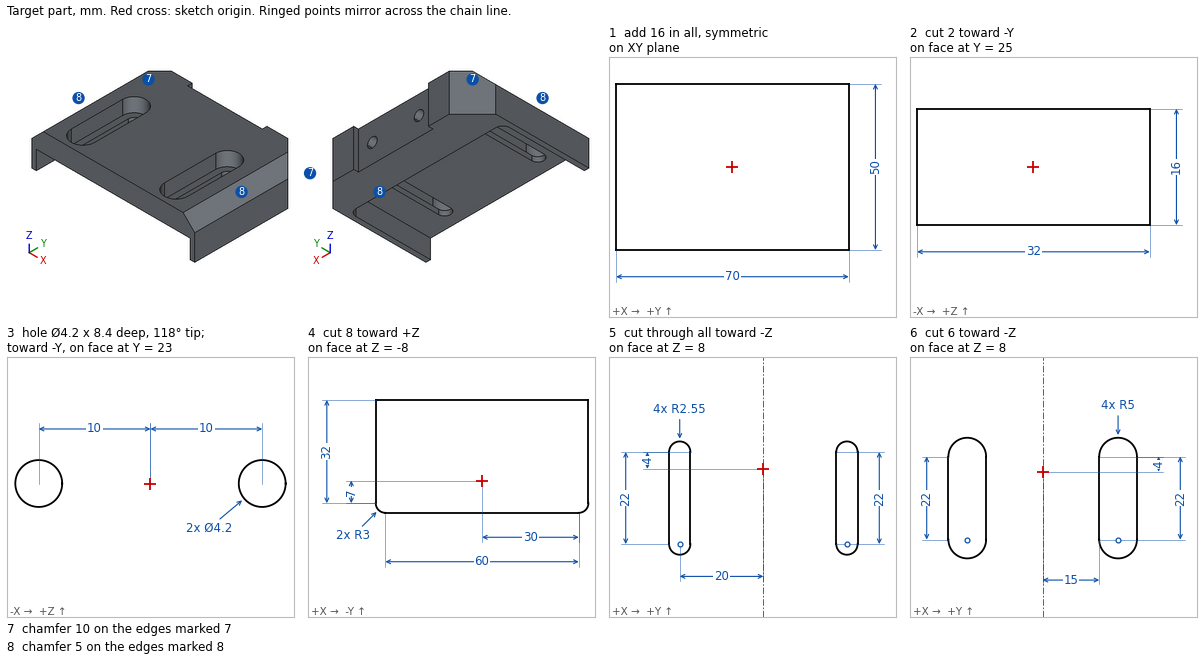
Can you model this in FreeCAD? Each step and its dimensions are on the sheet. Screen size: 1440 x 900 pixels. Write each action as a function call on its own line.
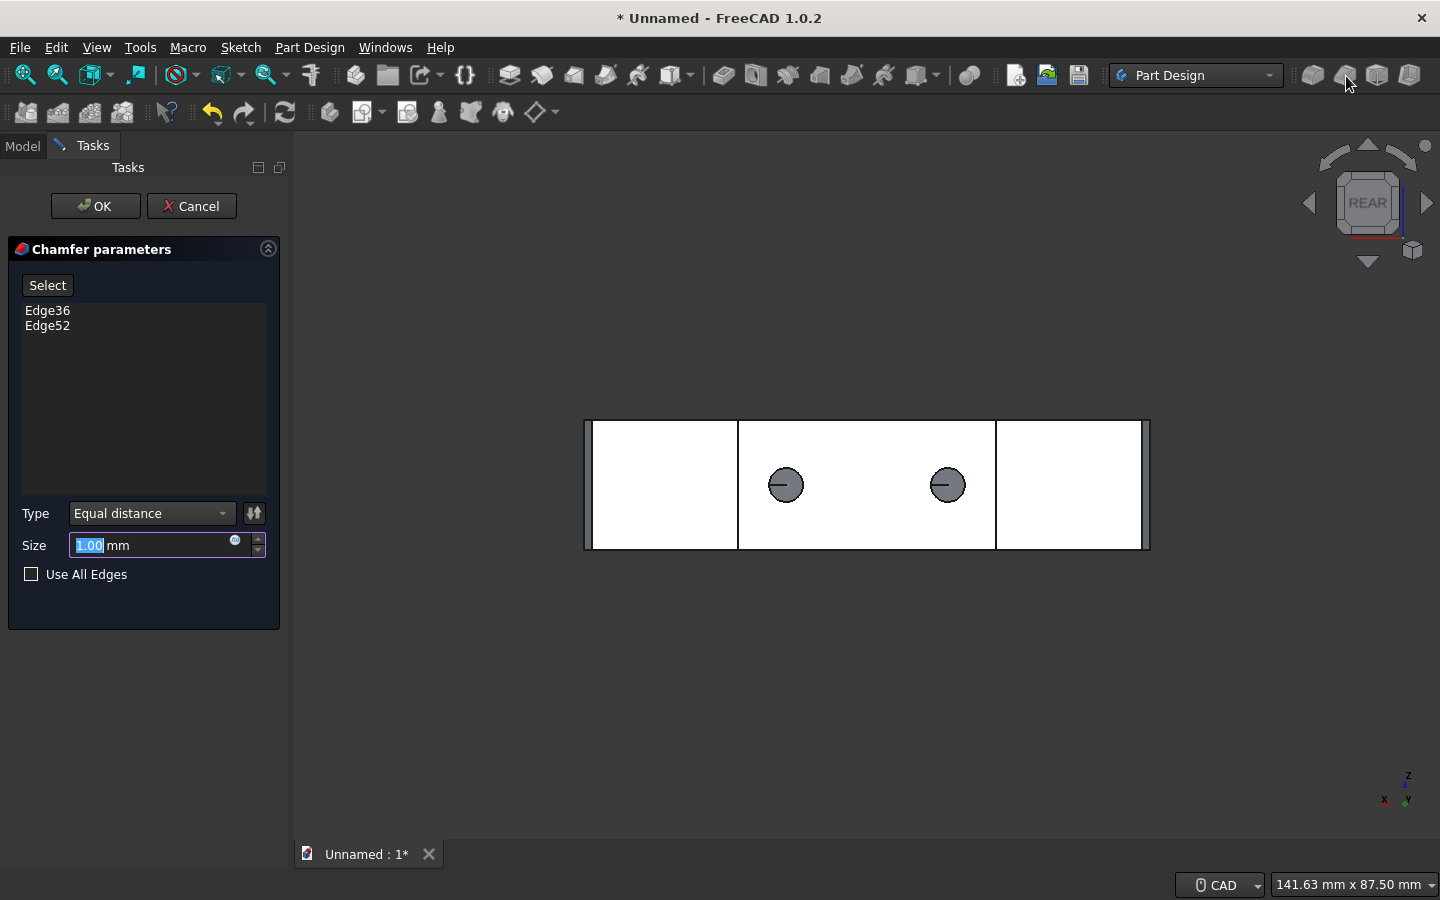
text(10)
key(Tab)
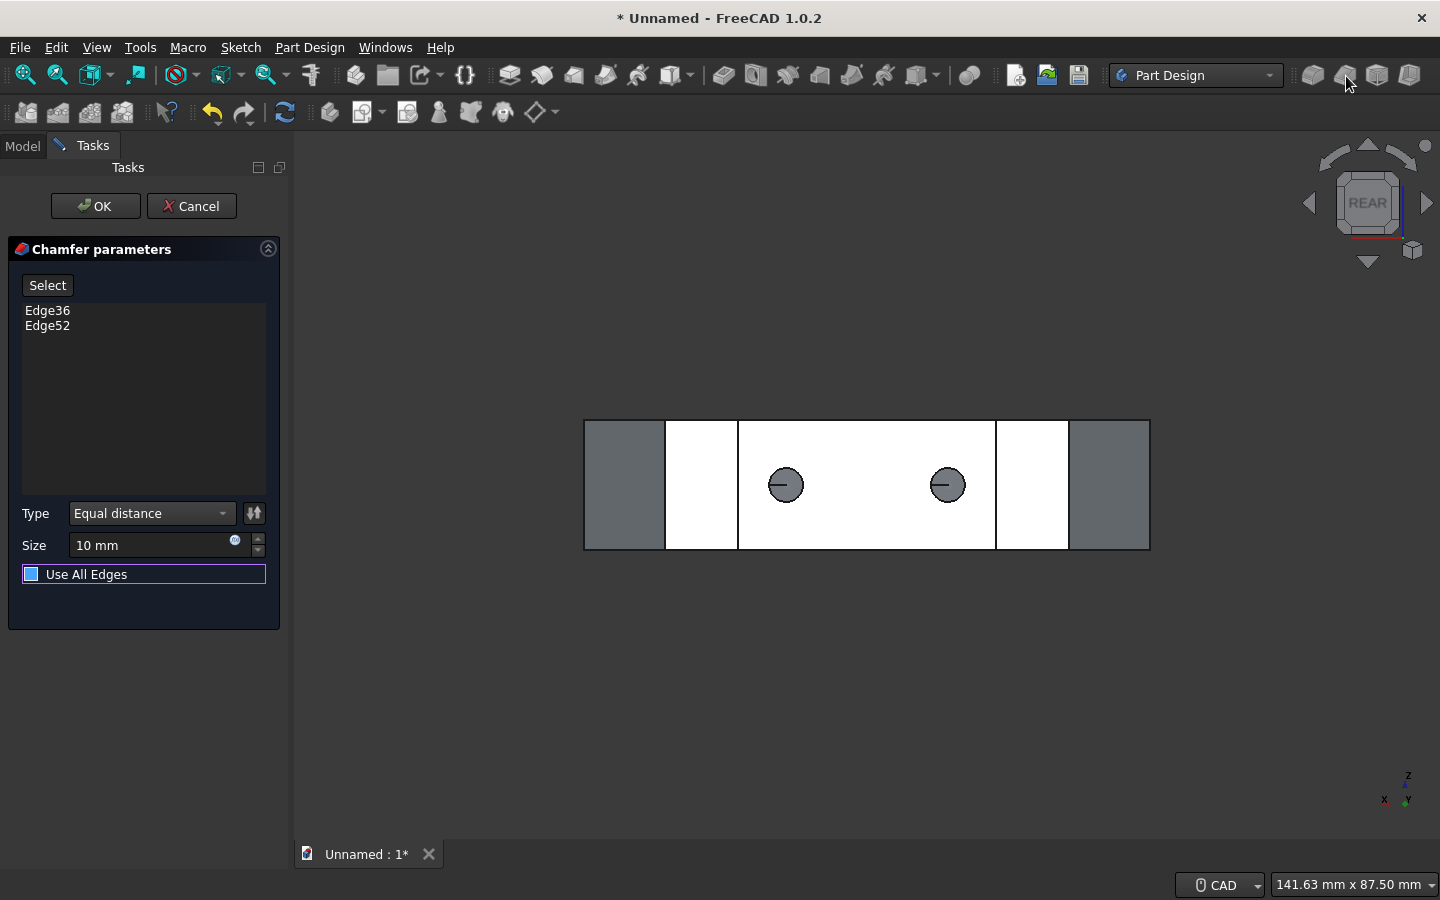
click(96, 206)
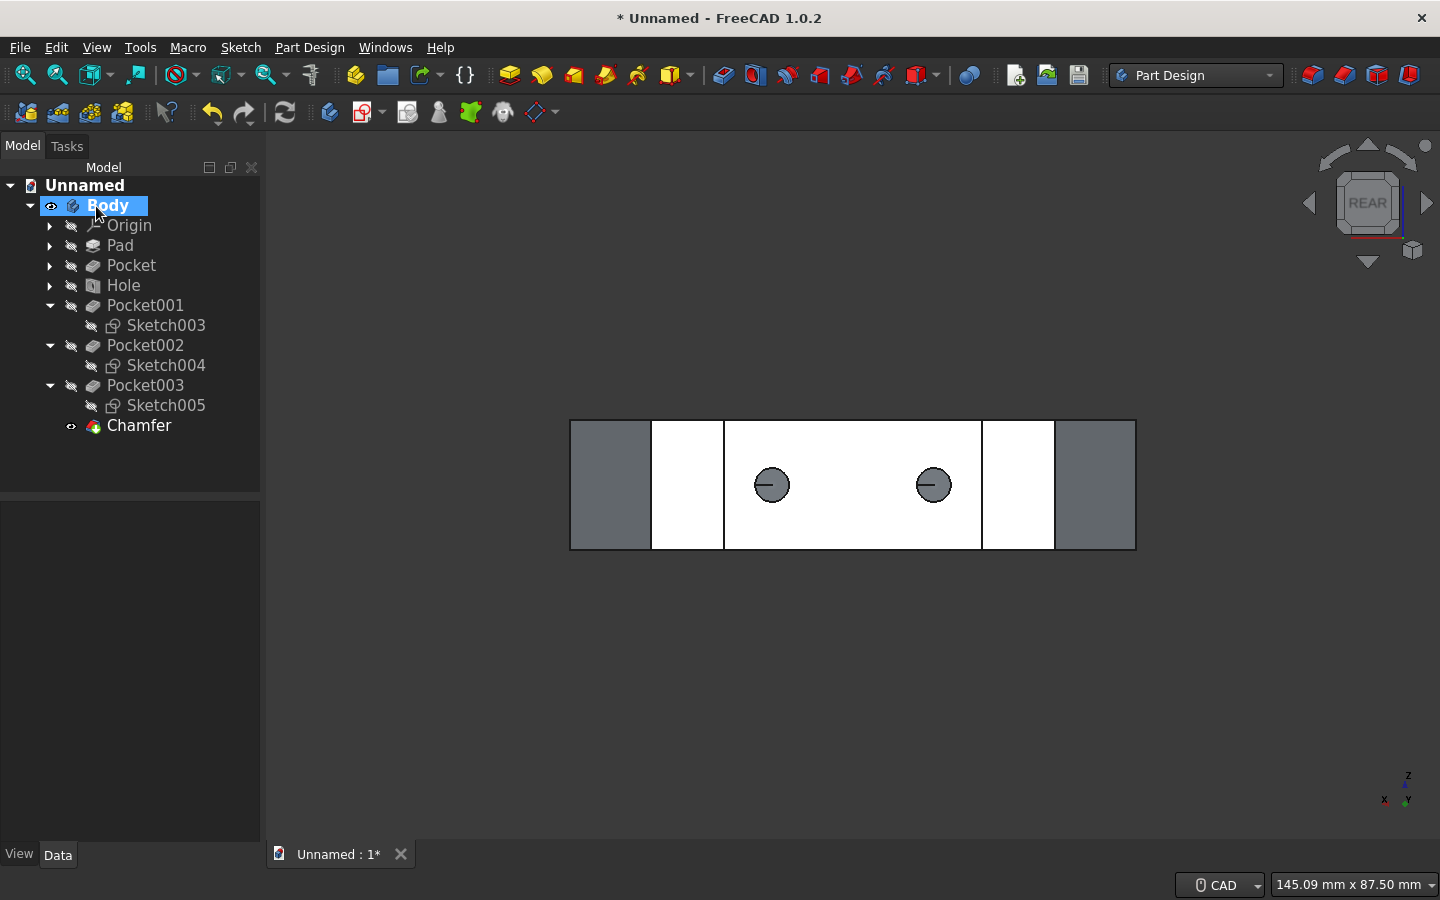
key(0)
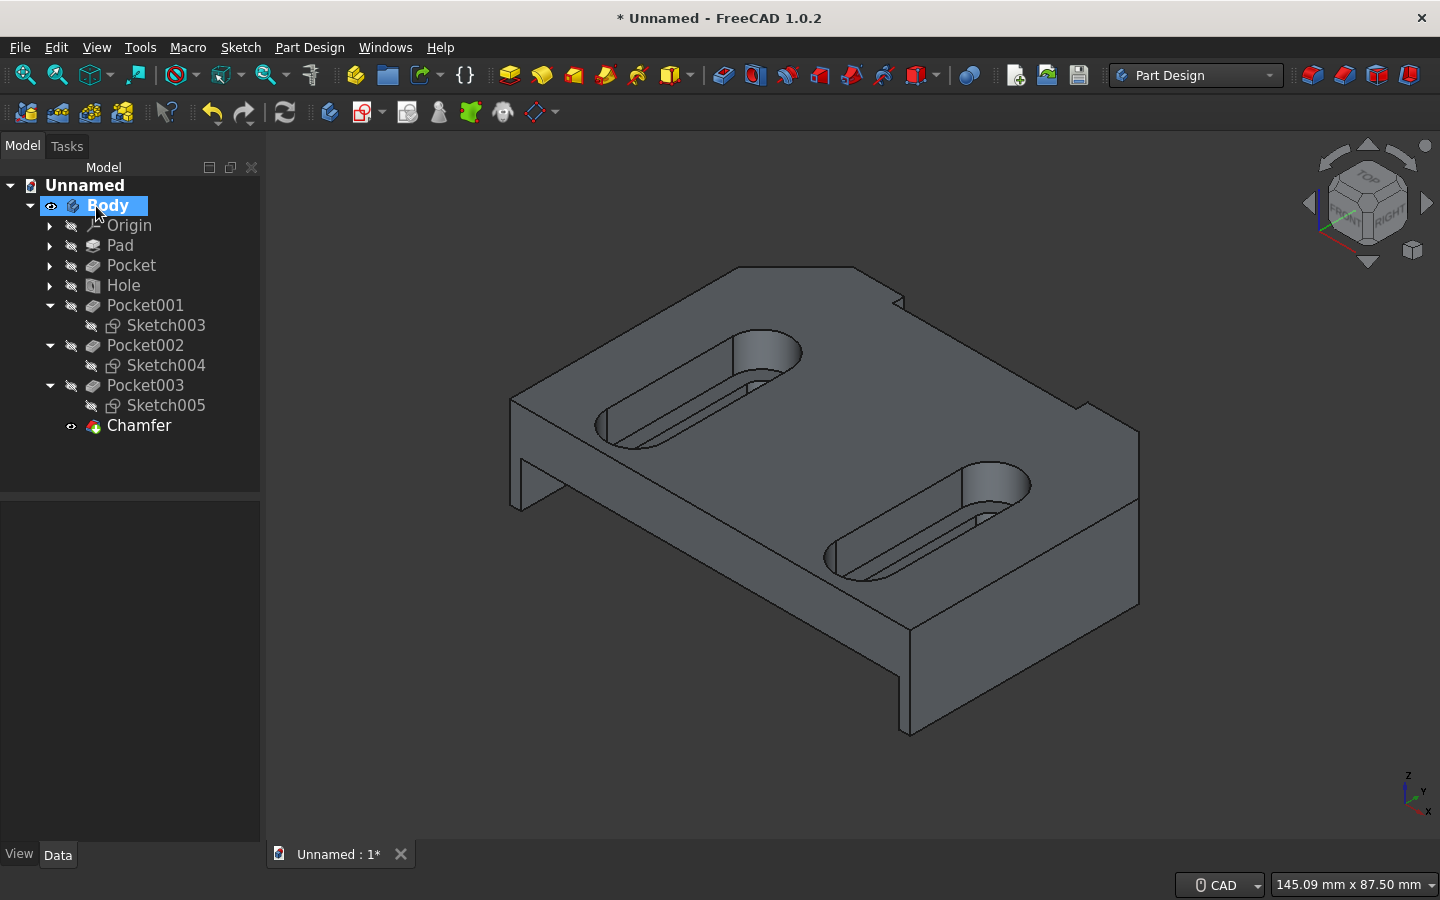
click(1025, 563)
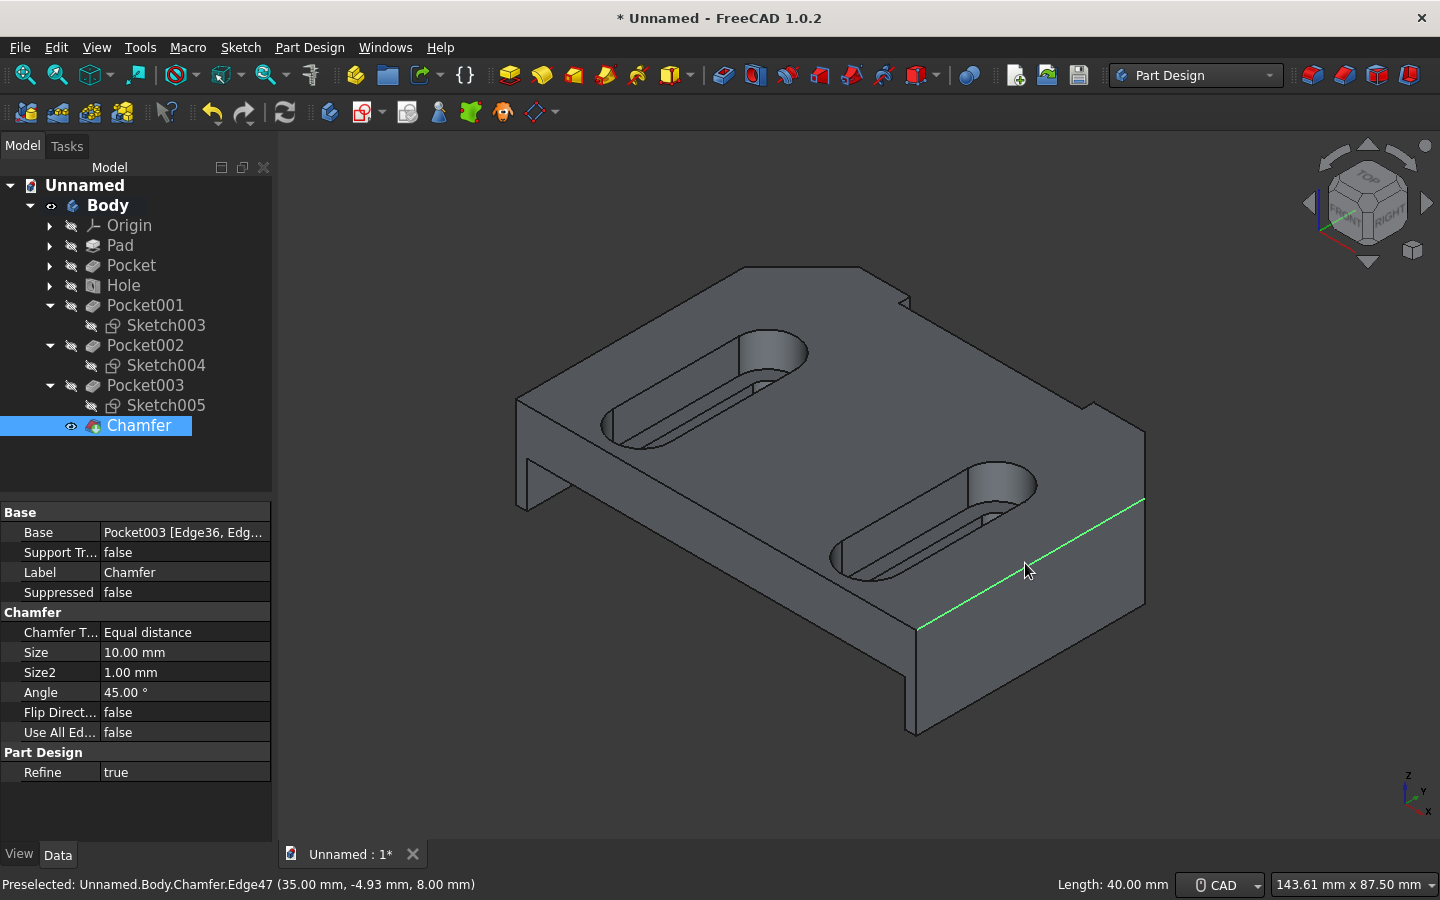
key(2)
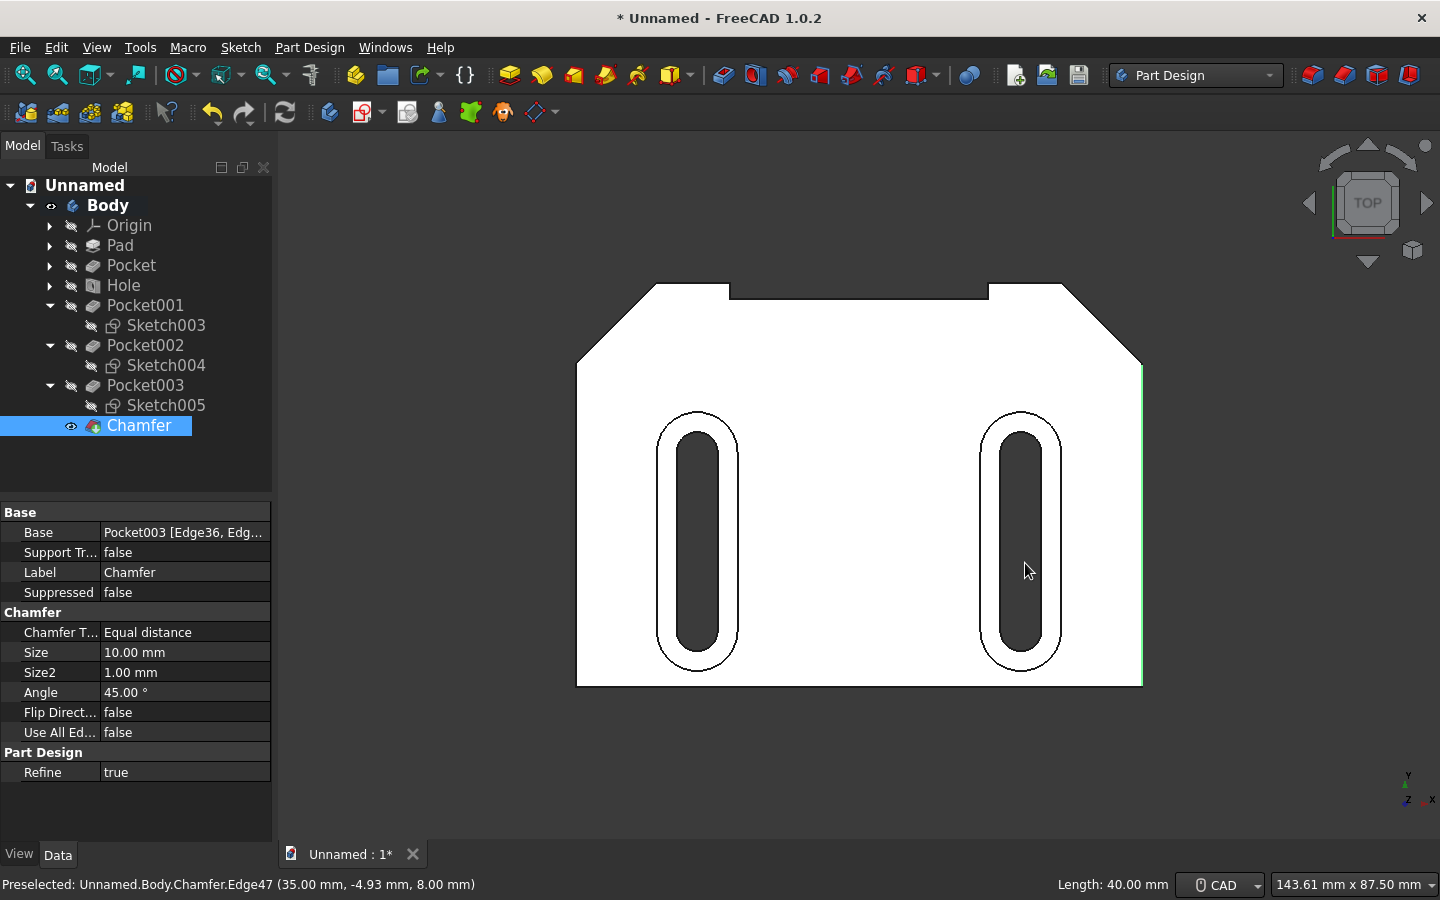
click(576, 524, ctrl)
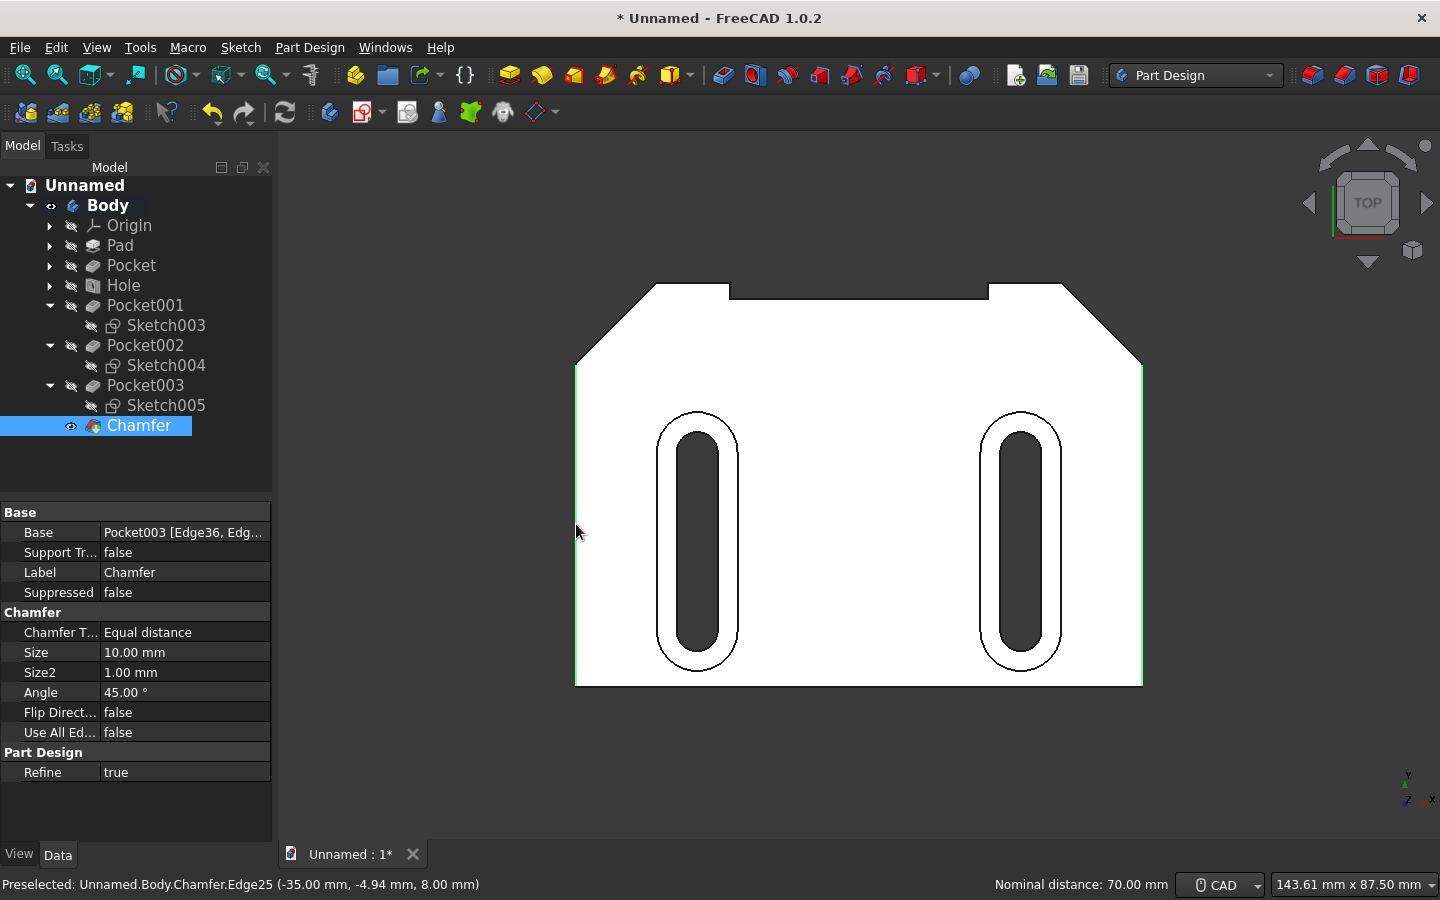
click(1346, 76)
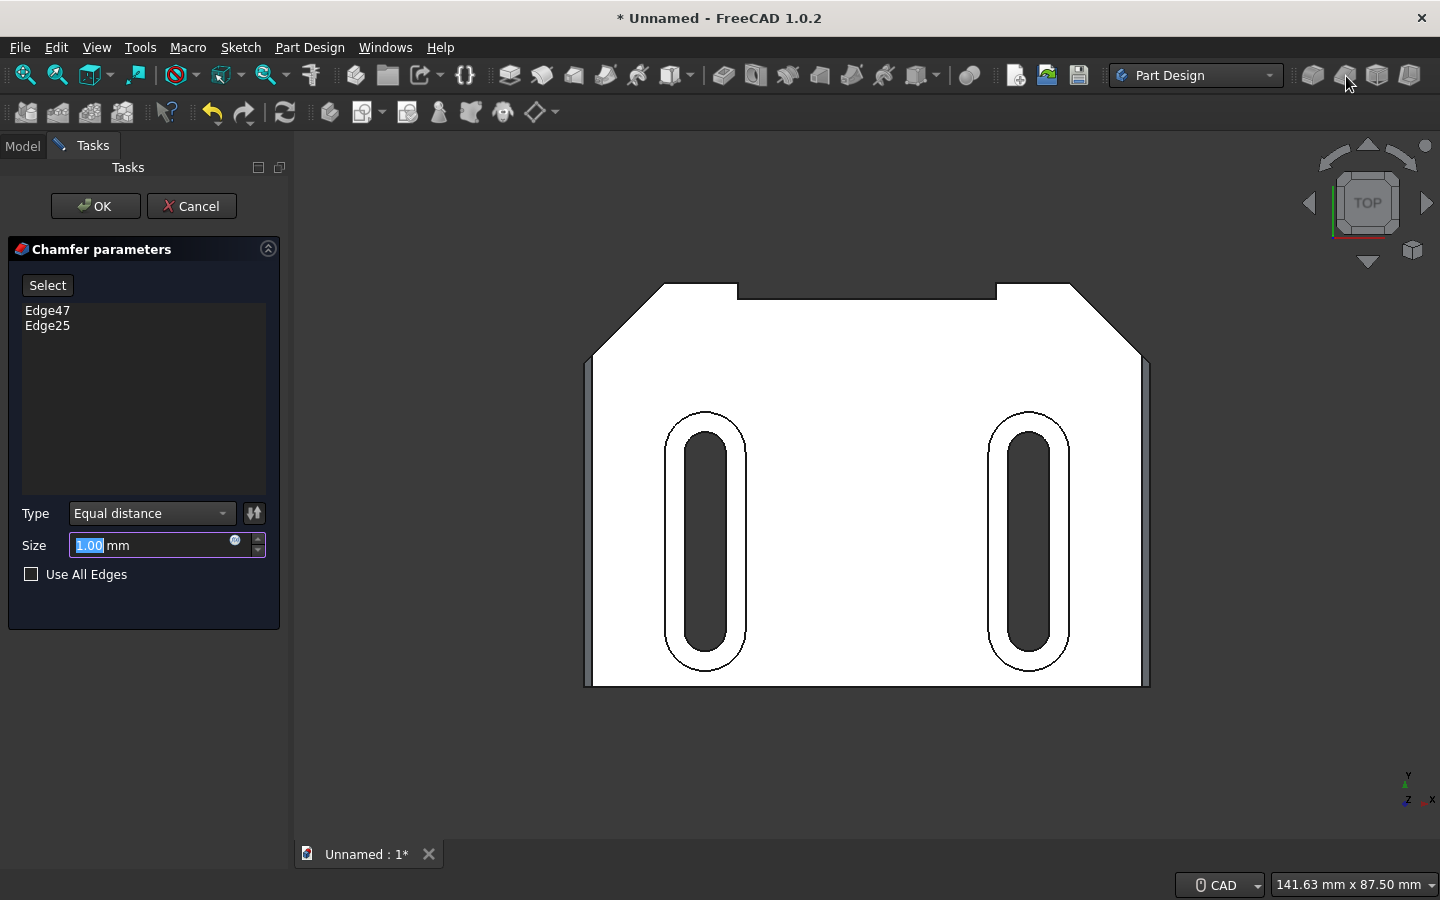
text(5)
key(Tab)